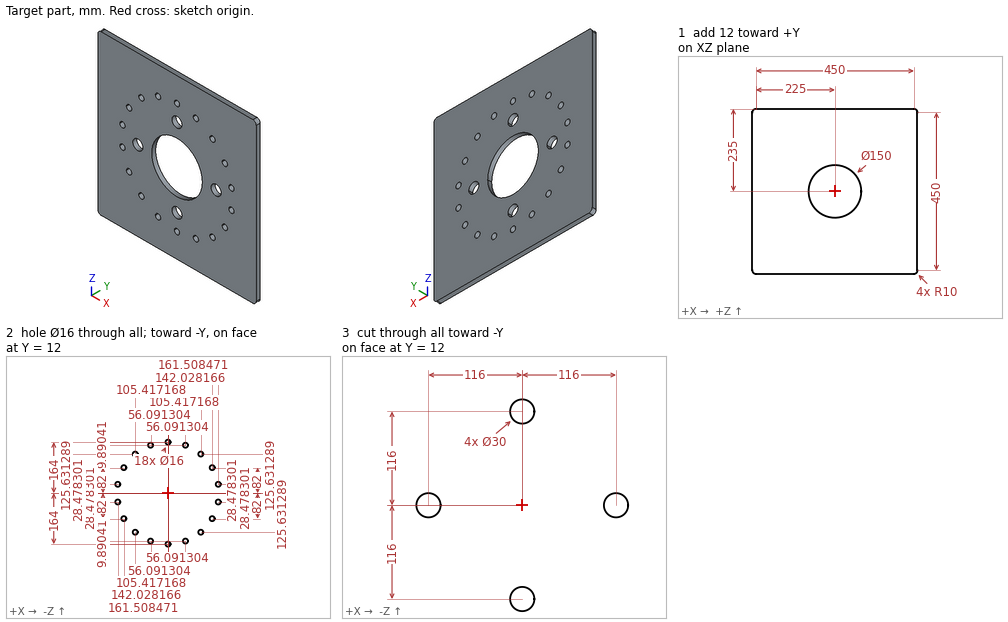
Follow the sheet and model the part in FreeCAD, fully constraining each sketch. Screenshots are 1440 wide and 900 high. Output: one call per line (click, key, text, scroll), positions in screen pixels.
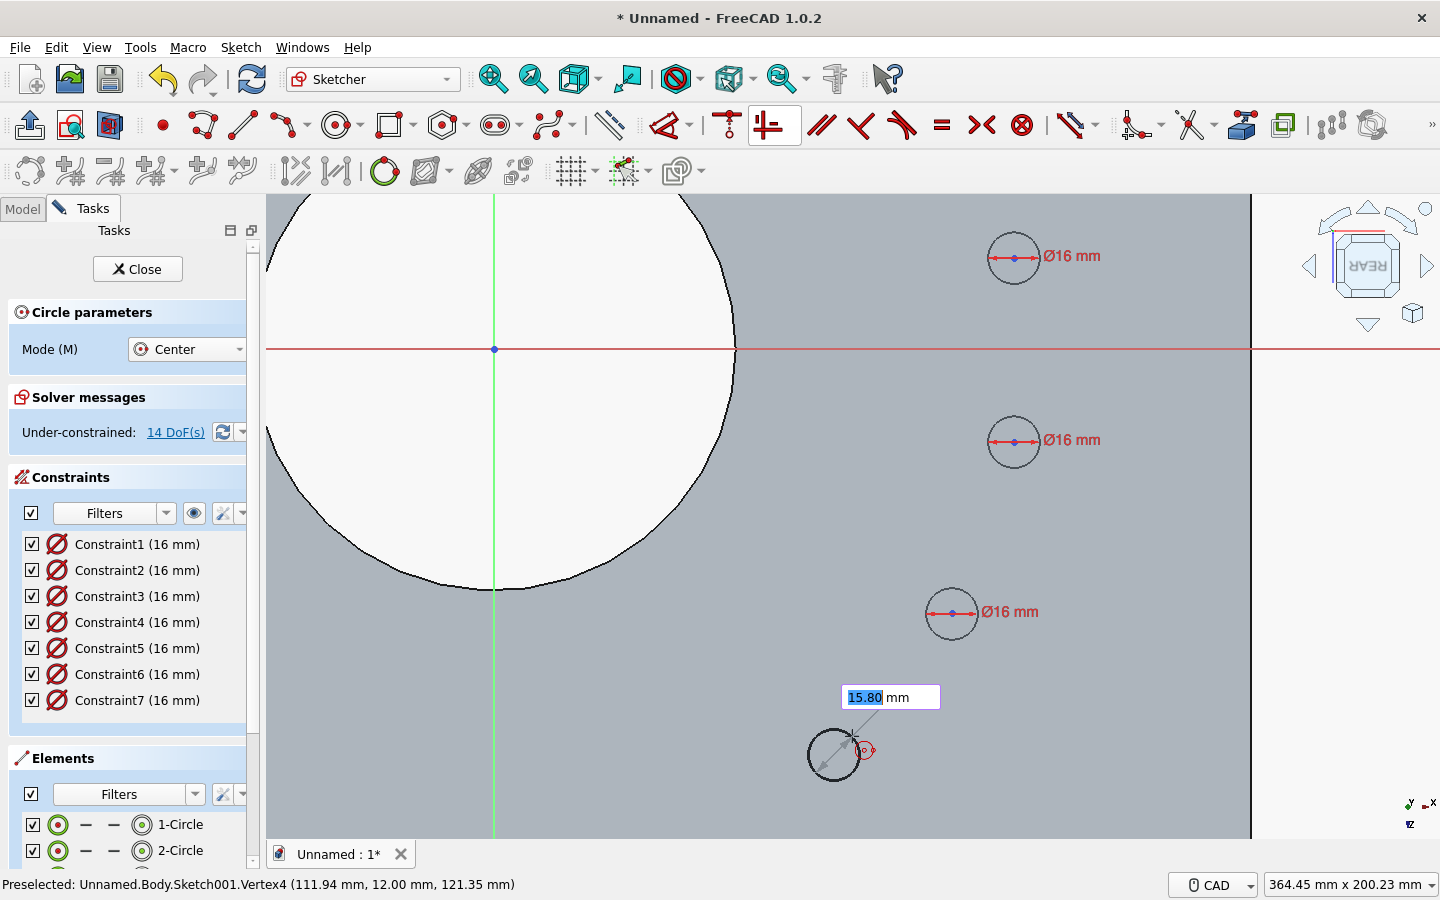
text(16)
key(Return)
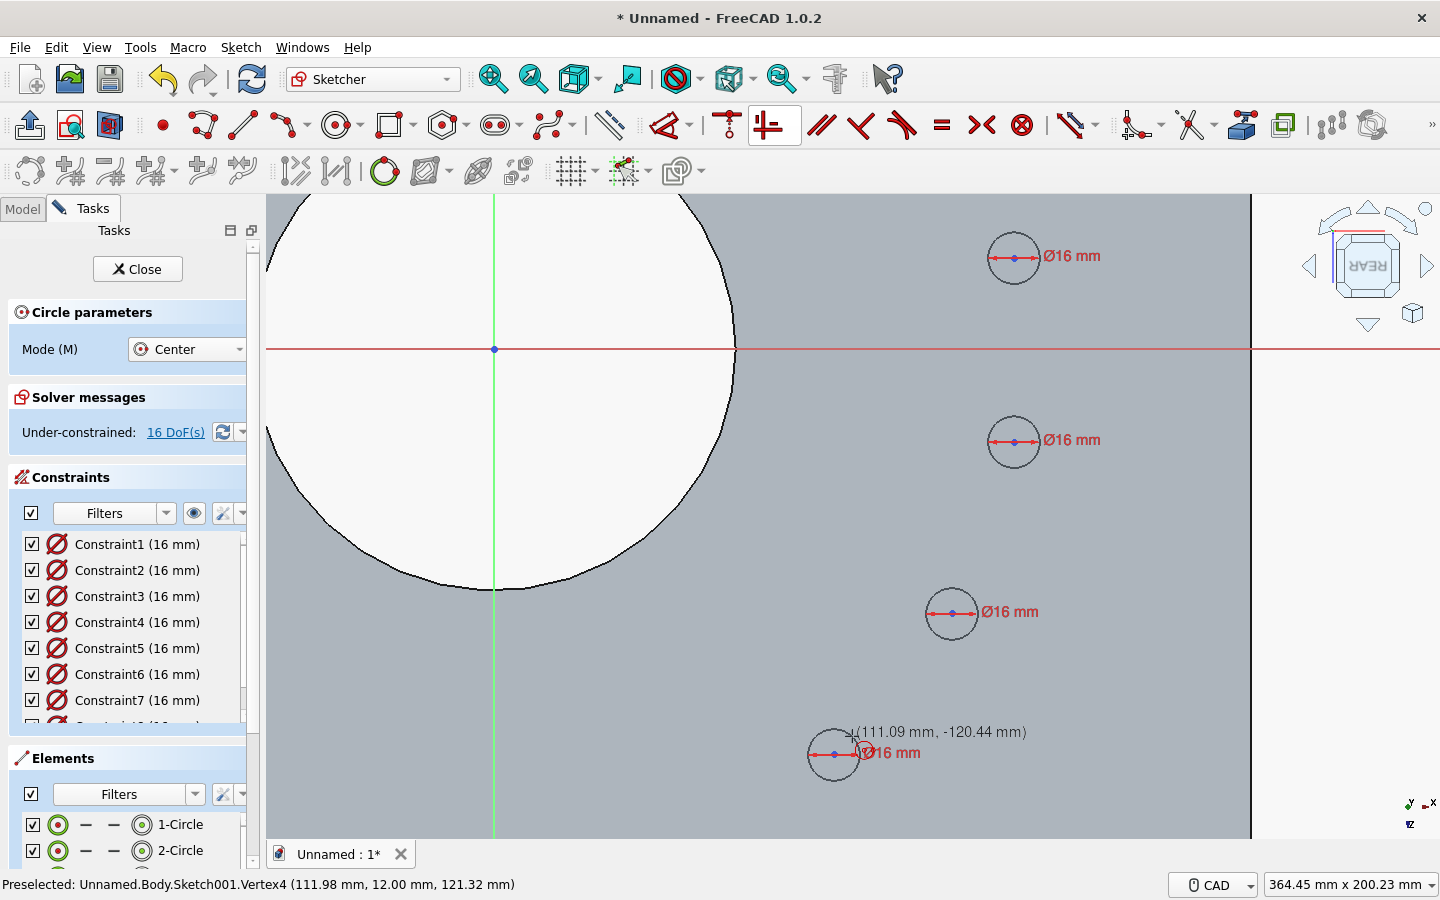
scroll(953, 614, down, 5)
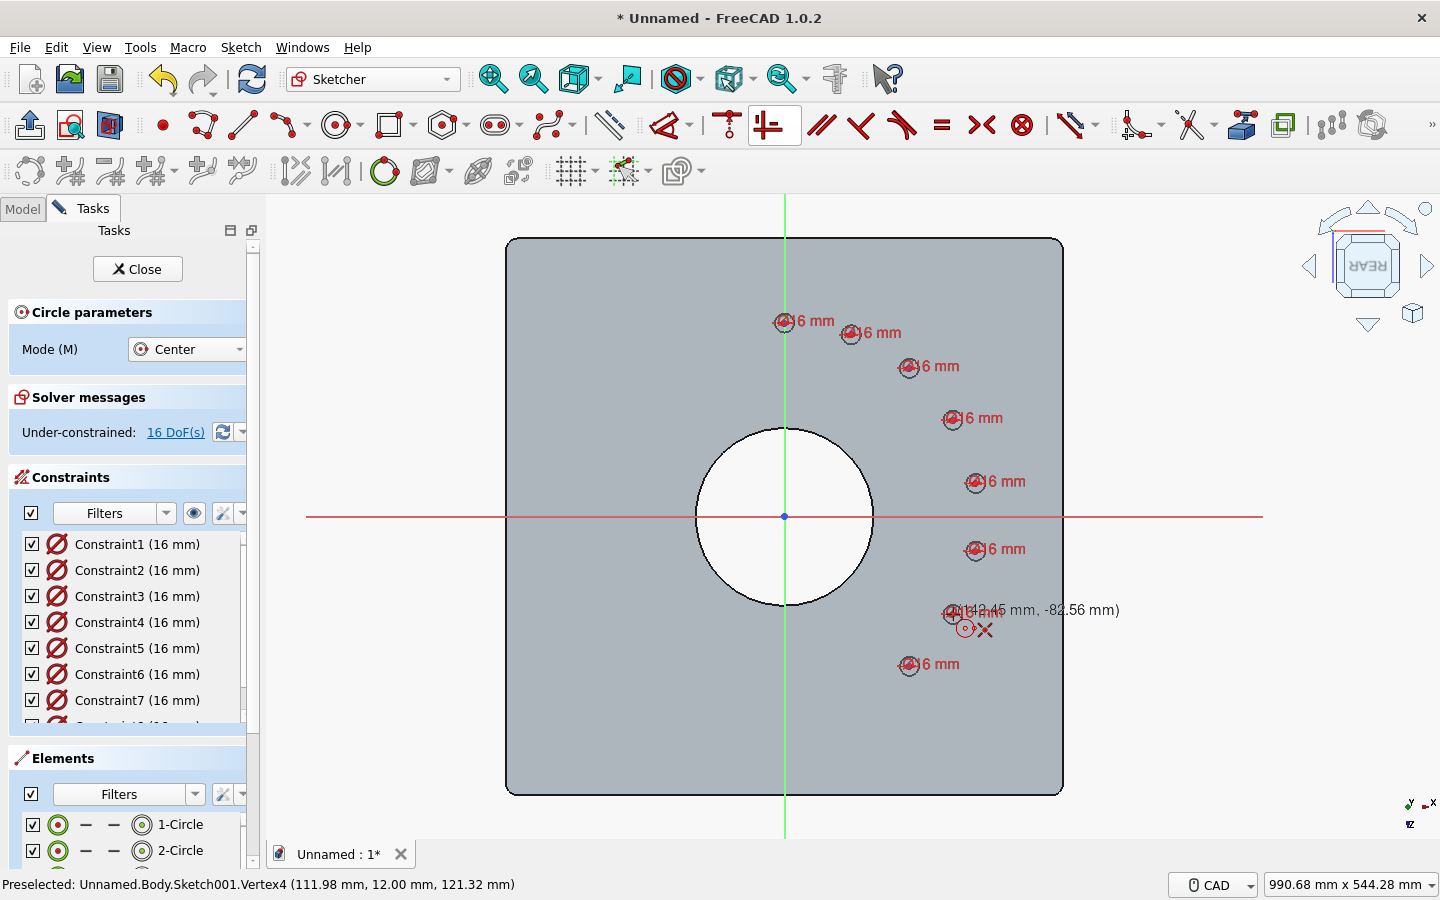
scroll(851, 700, up, 5)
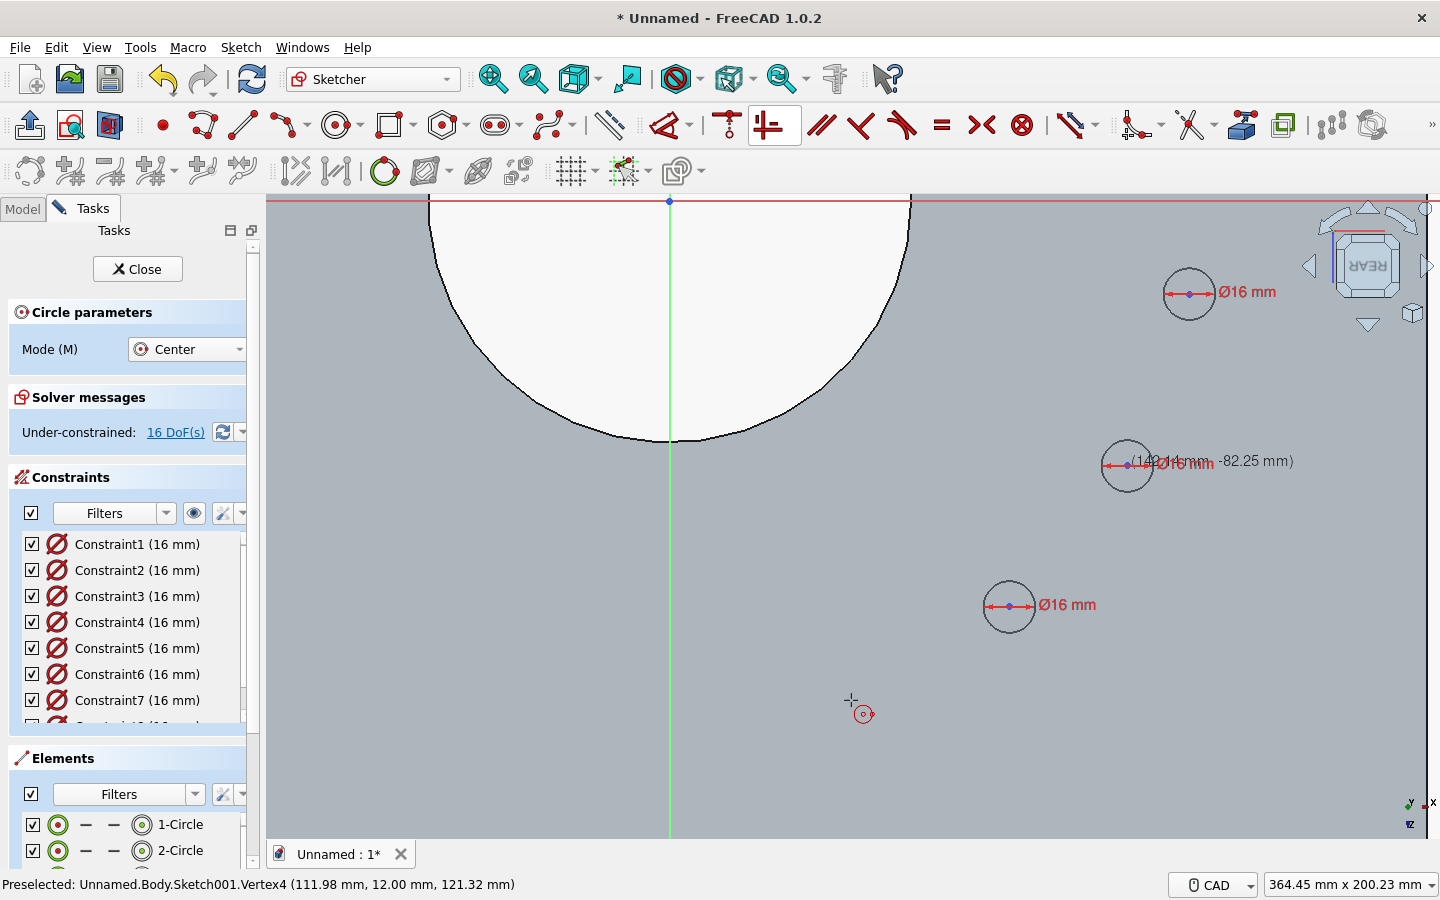
click(850, 697)
move(868, 679)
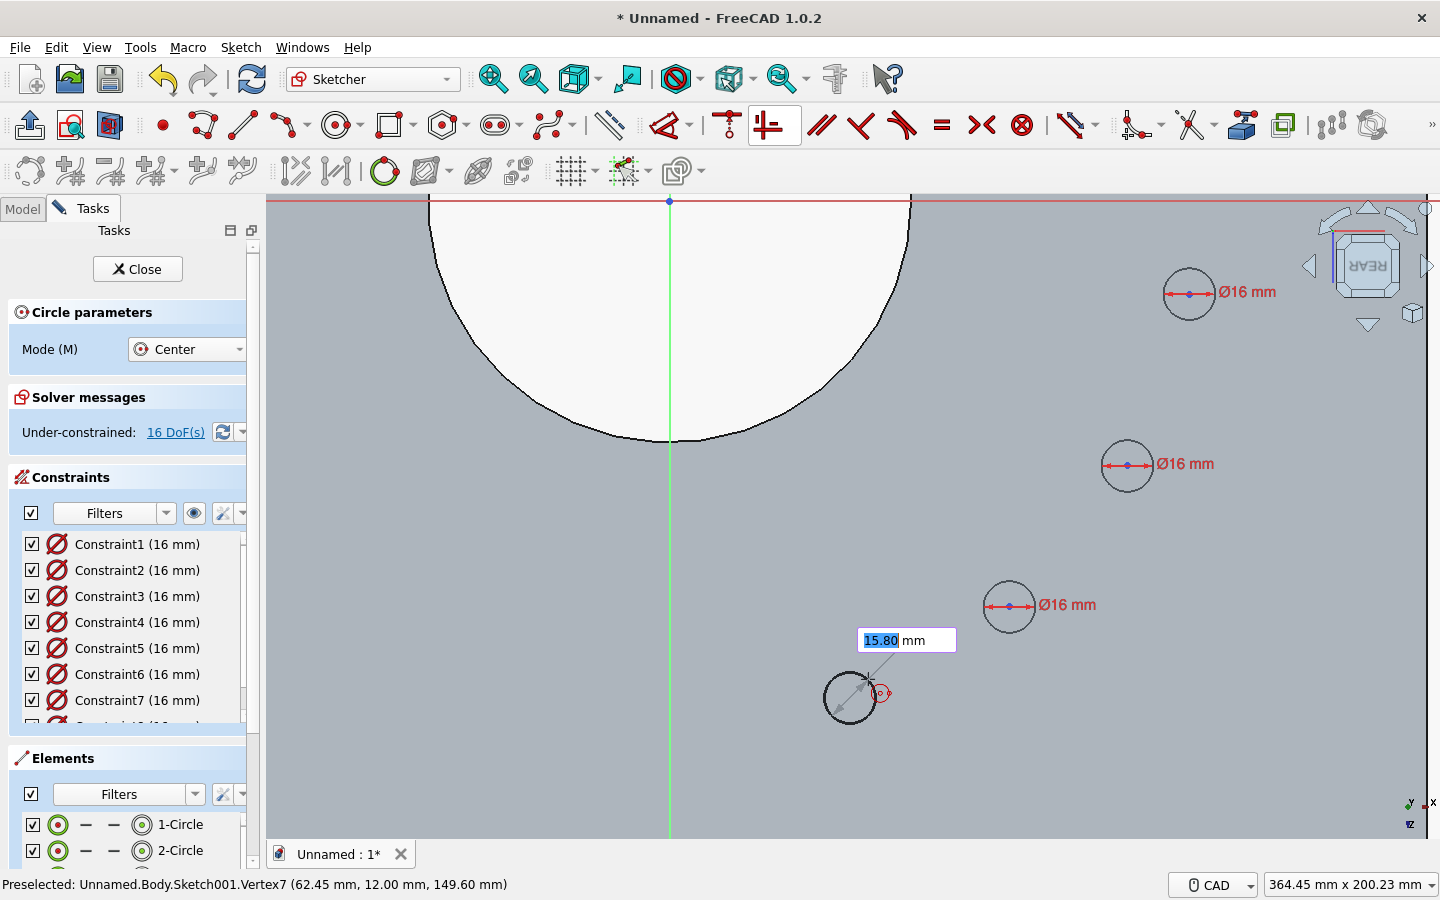
text(16)
key(Return)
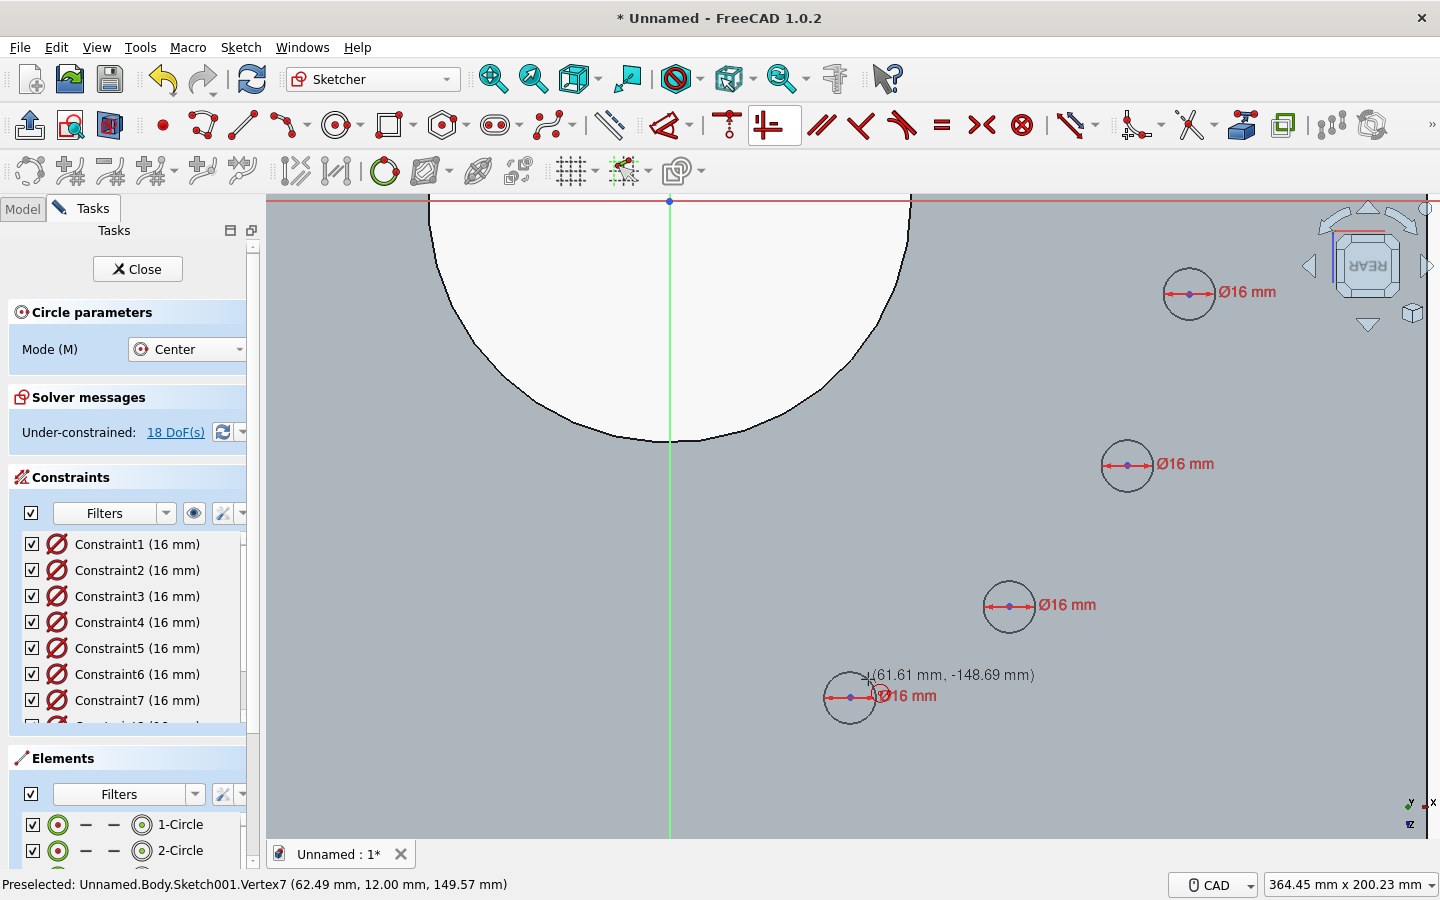
click(670, 729)
move(688, 711)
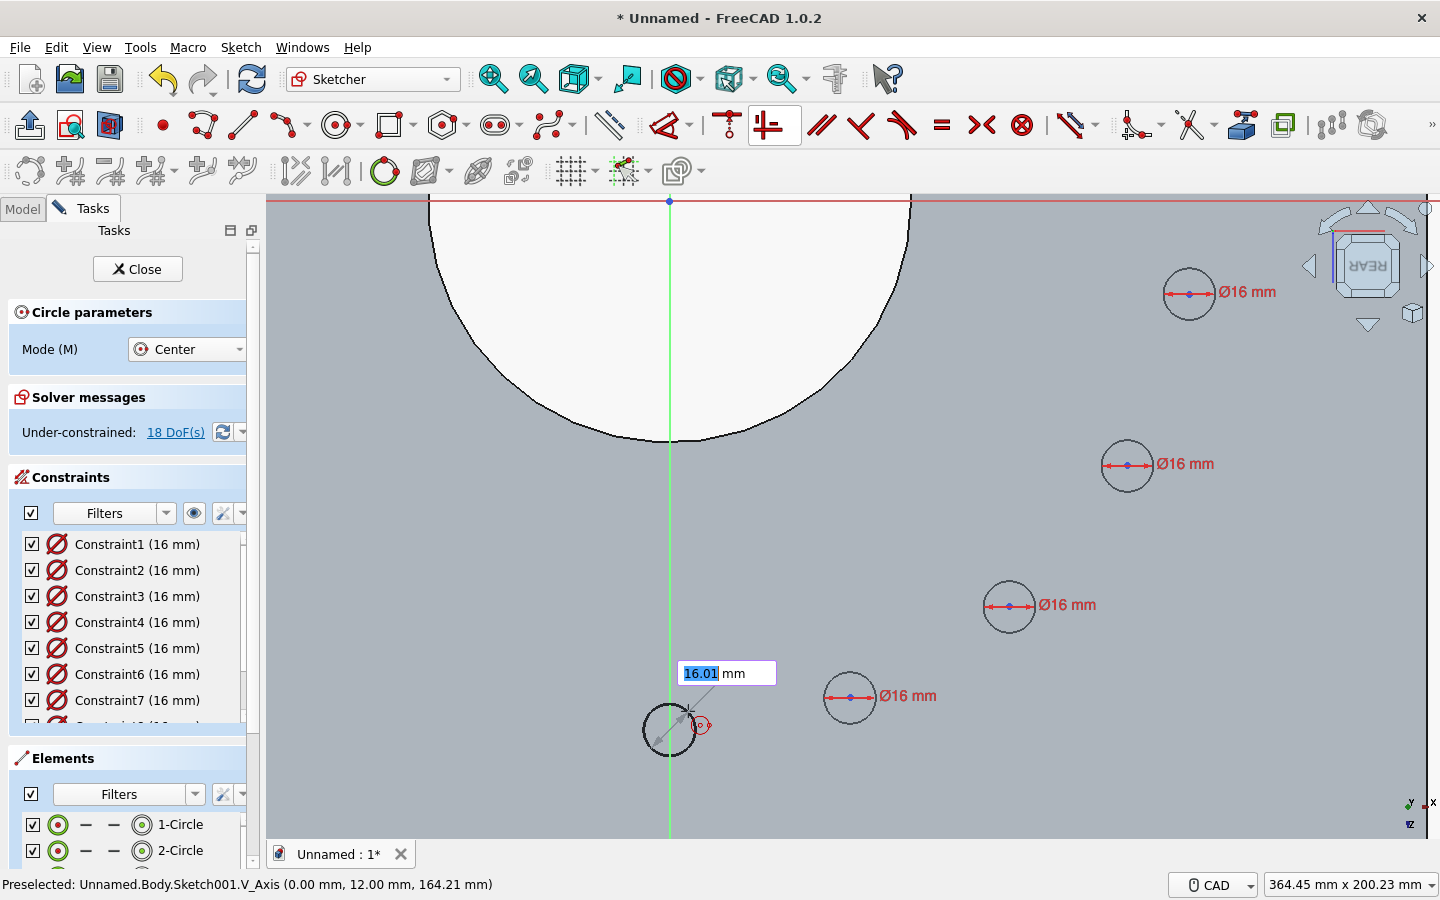
text(16)
key(Return)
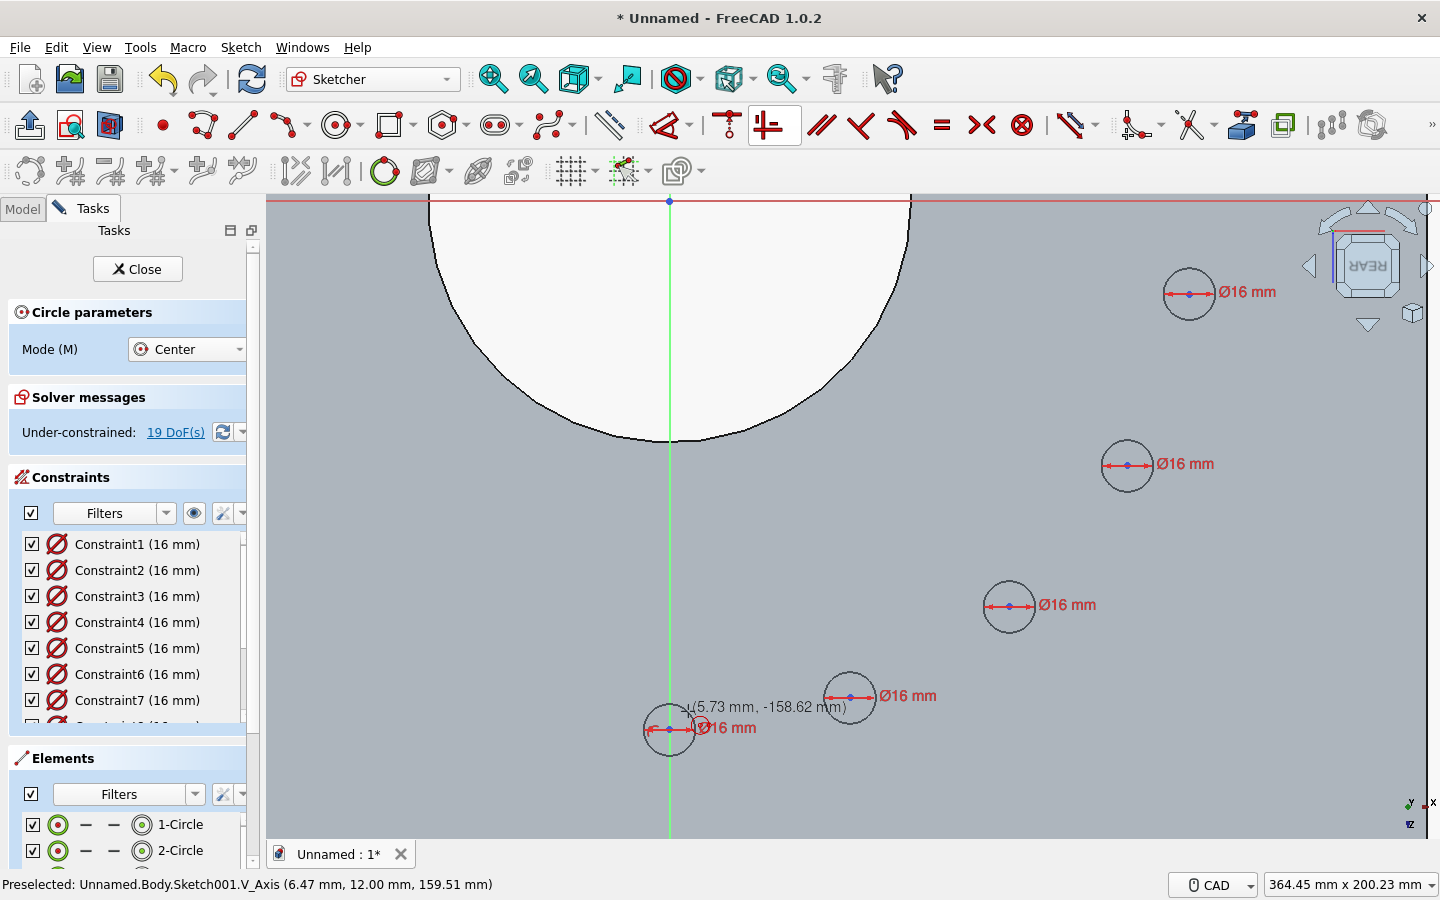
click(489, 697)
move(507, 679)